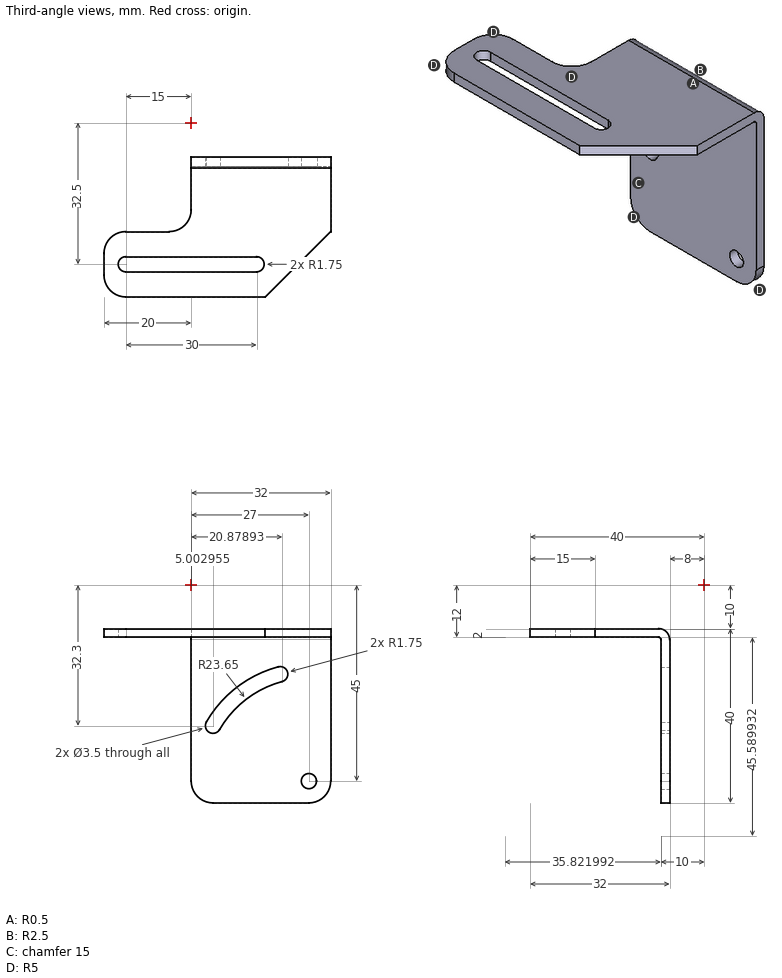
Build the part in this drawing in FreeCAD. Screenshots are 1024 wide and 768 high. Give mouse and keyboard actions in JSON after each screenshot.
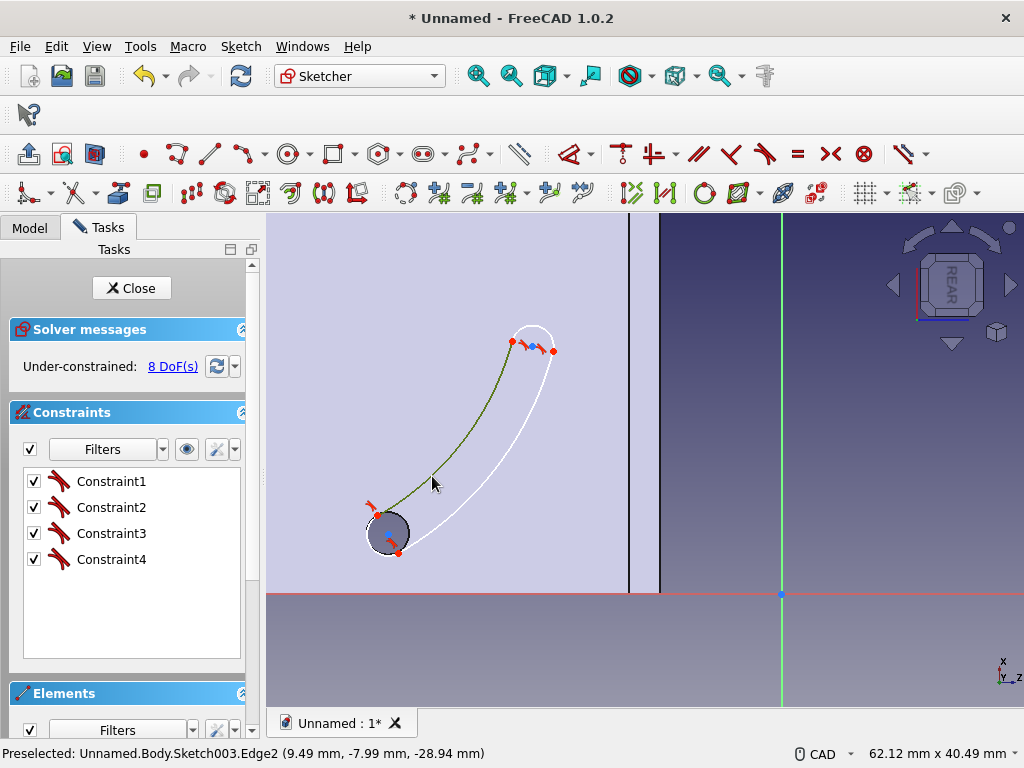
{"action": "left_click", "coordinate": [461, 506]}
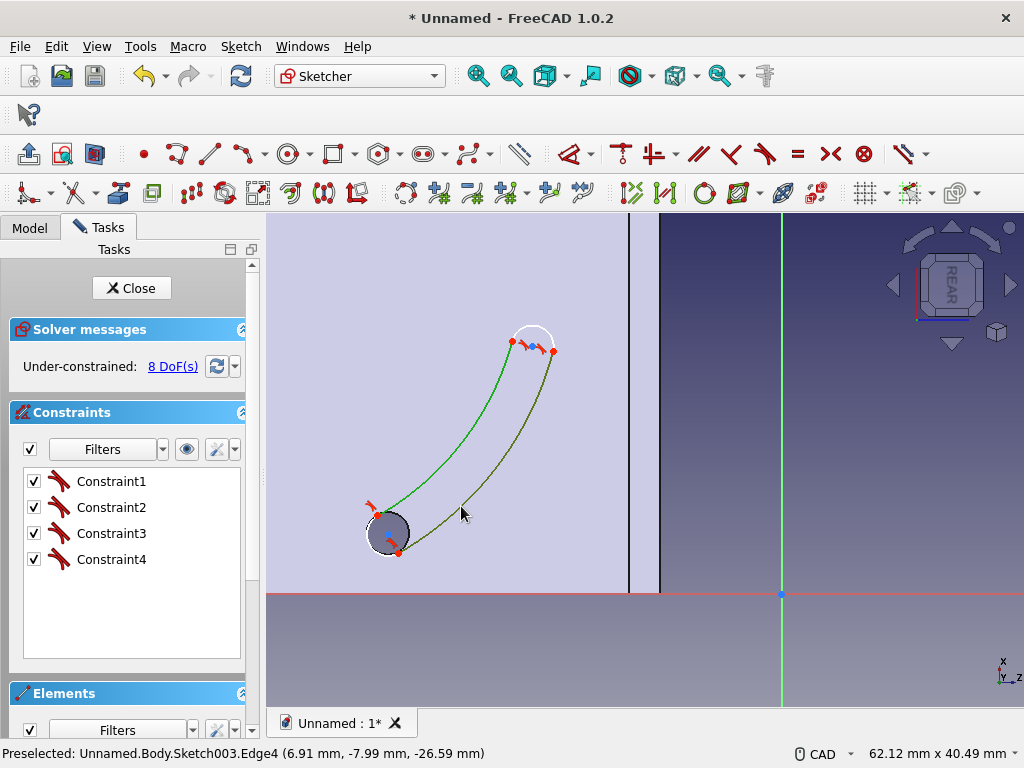
{"action": "key", "text": "c"}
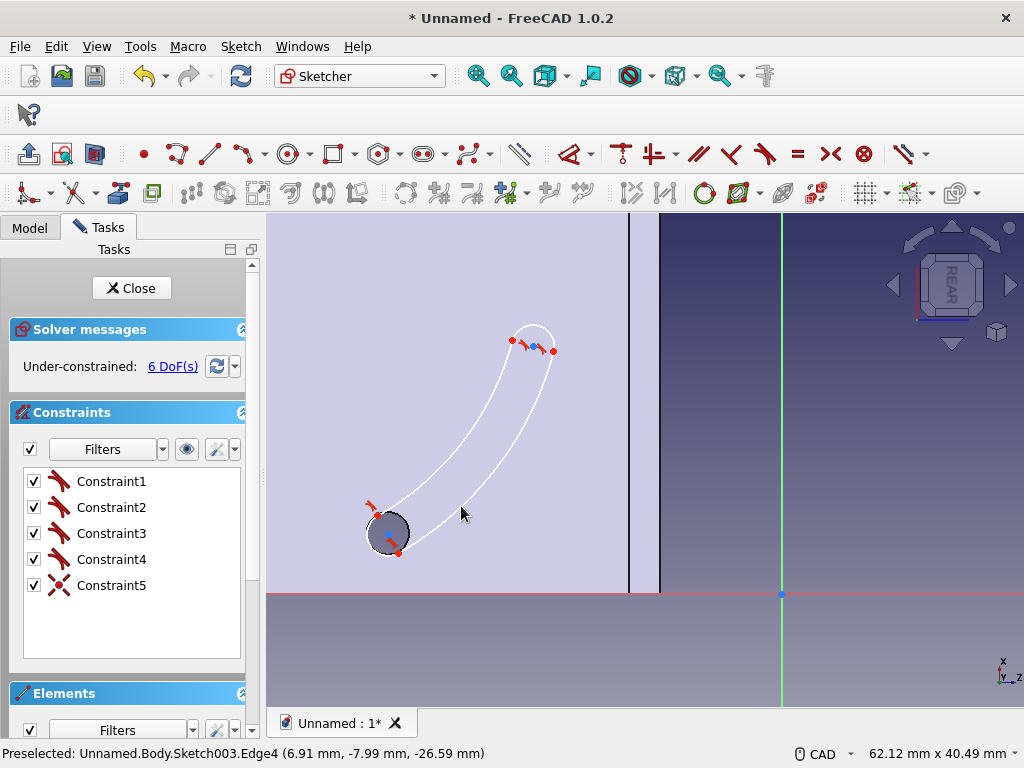
{"action": "key", "text": "d"}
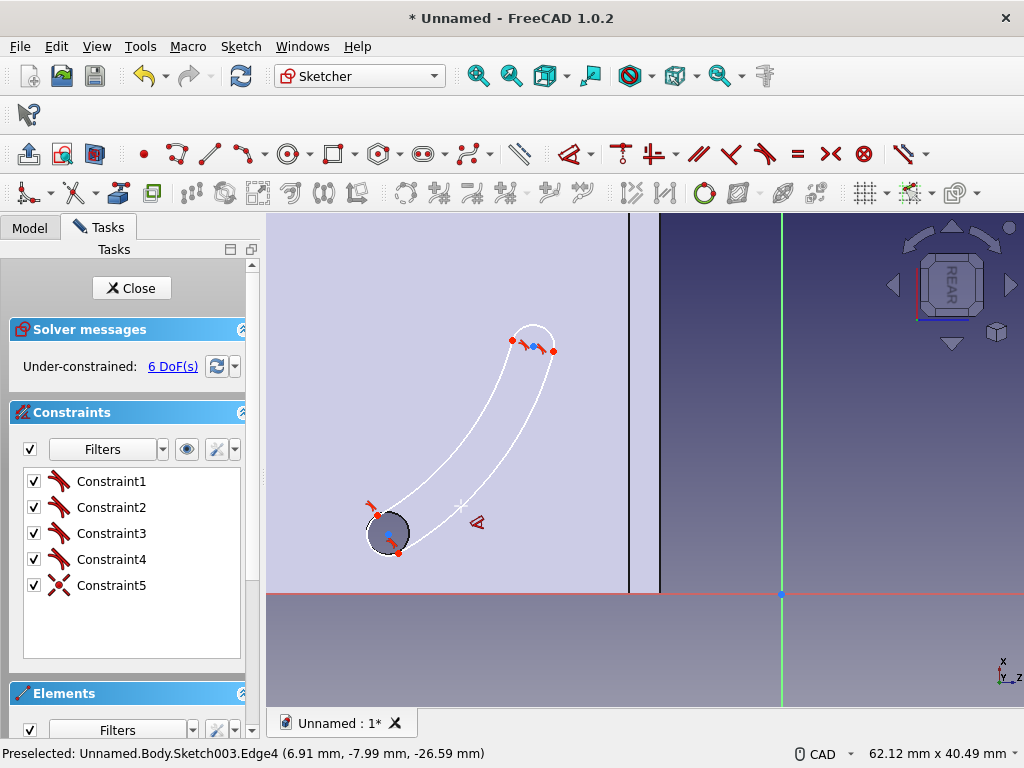
{"action": "scroll", "coordinate": [550, 333], "scroll_direction": "up", "scroll_amount": 4}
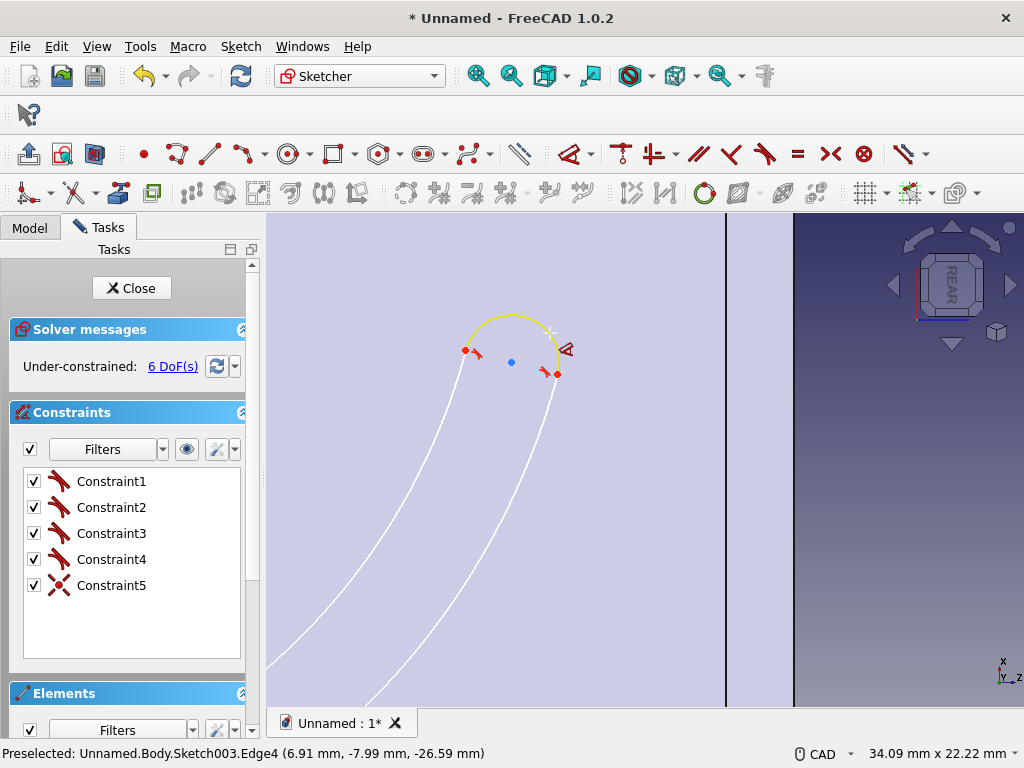
{"action": "left_click", "coordinate": [549, 333]}
{"action": "left_click", "coordinate": [574, 313]}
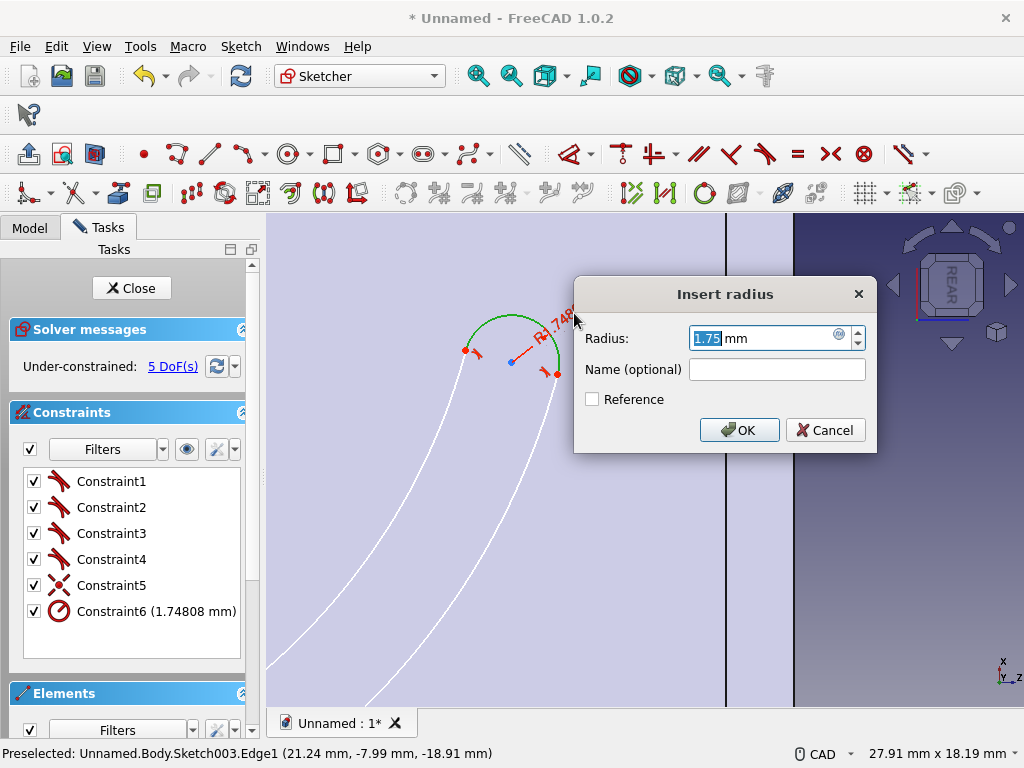
{"action": "type", "text": "1.75"}
{"action": "key", "text": "Return"}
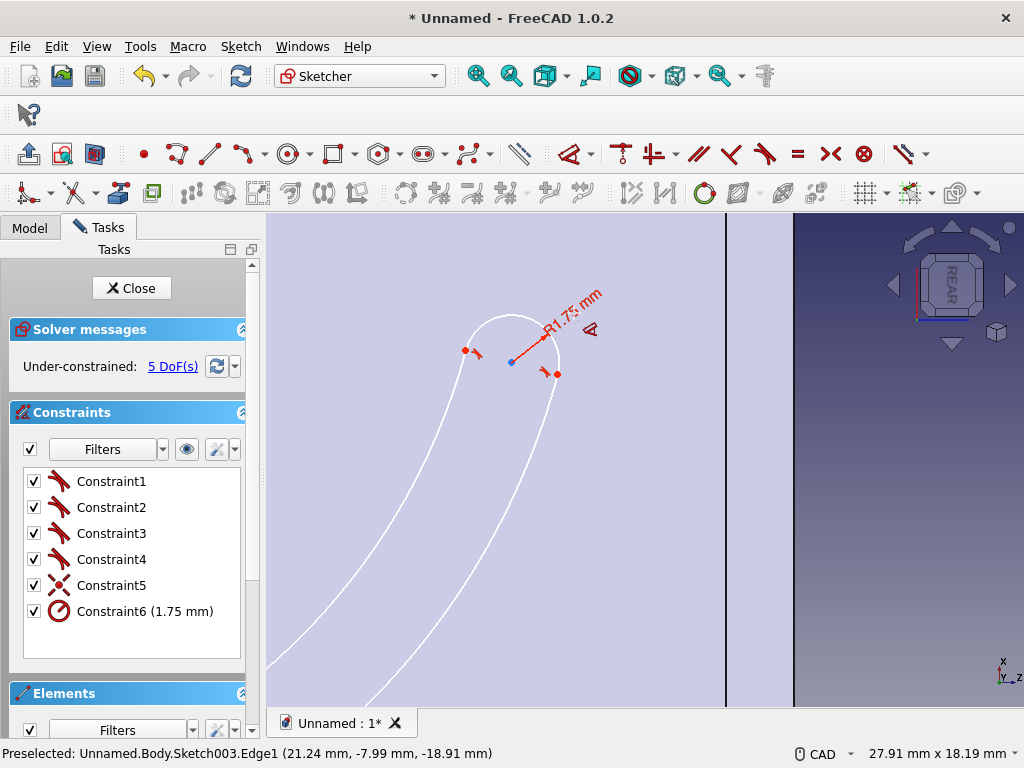
{"action": "left_click", "coordinate": [410, 491]}
{"action": "left_click", "coordinate": [438, 506]}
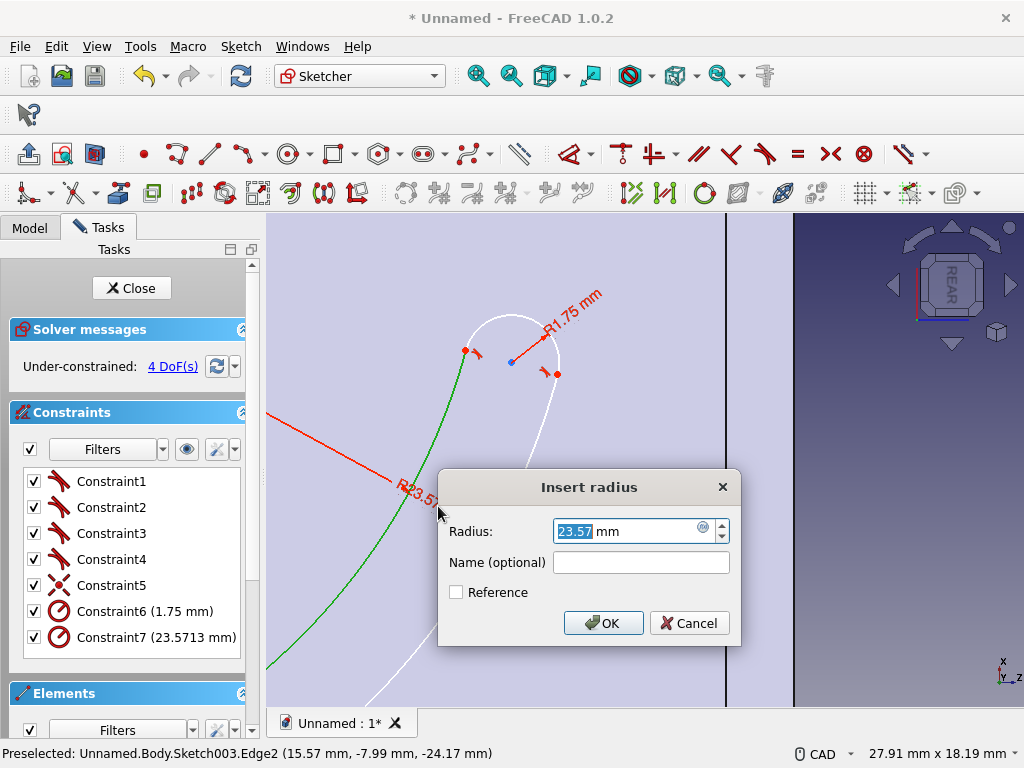
{"action": "type", "text": "23.65"}
{"action": "key", "text": "Return"}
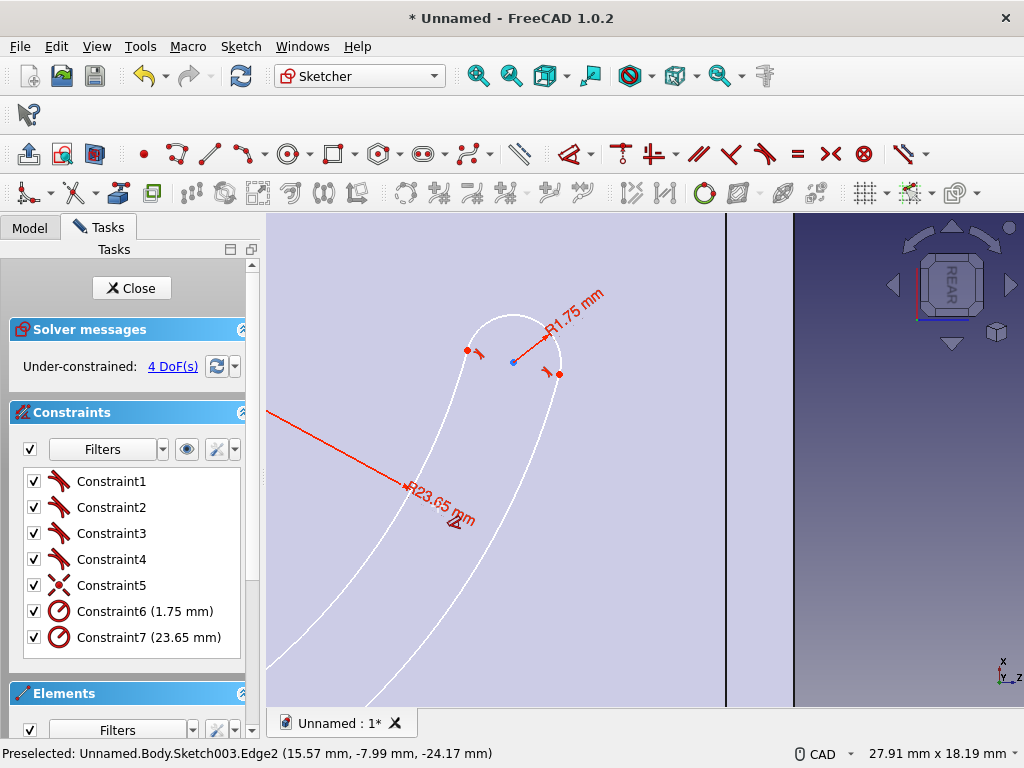
{"action": "scroll", "coordinate": [552, 334], "scroll_direction": "down", "scroll_amount": 4}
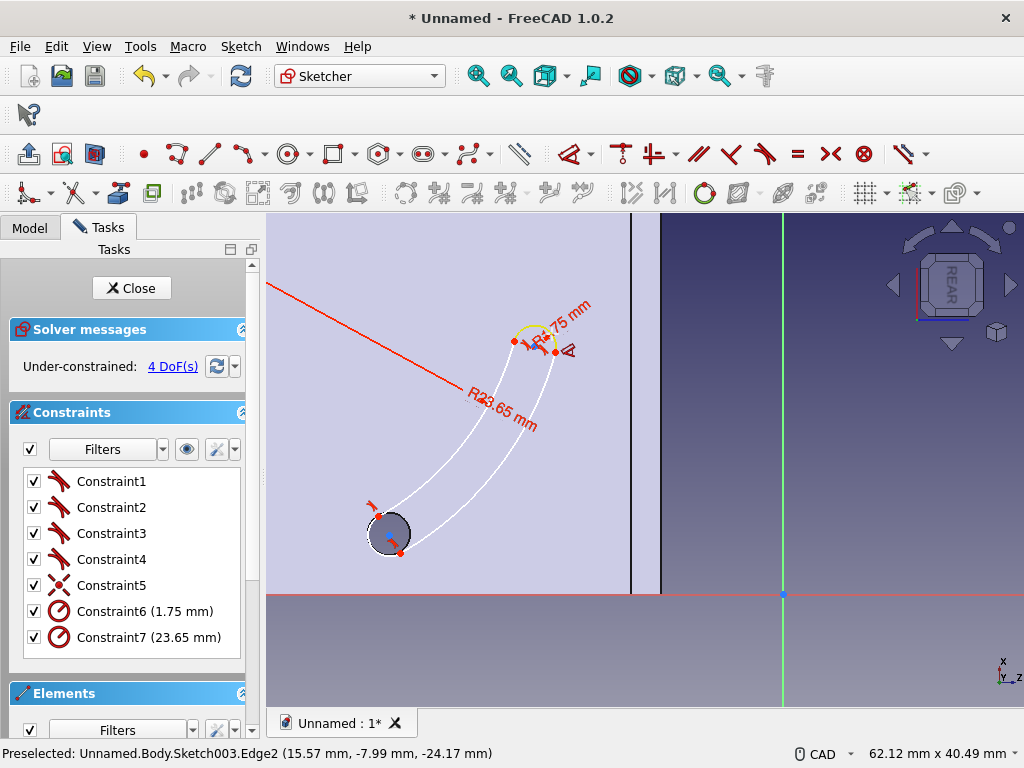
{"action": "scroll", "coordinate": [713, 520], "scroll_direction": "down", "scroll_amount": 2}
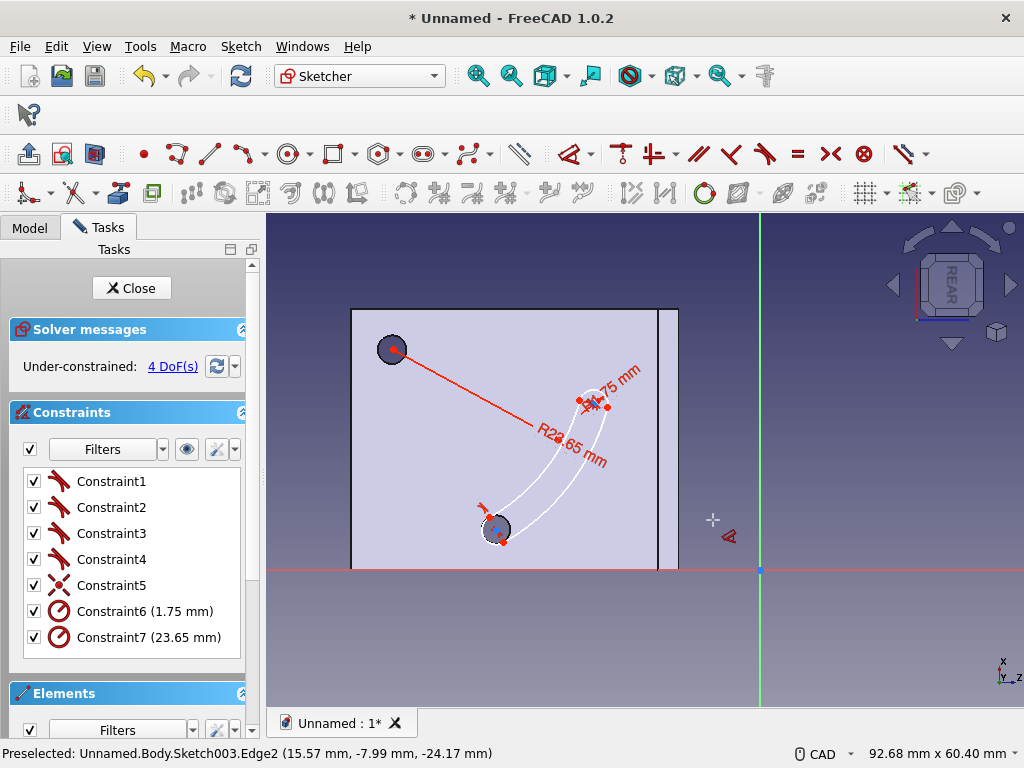
{"action": "left_click", "coordinate": [393, 350]}
{"action": "left_click", "coordinate": [577, 316]}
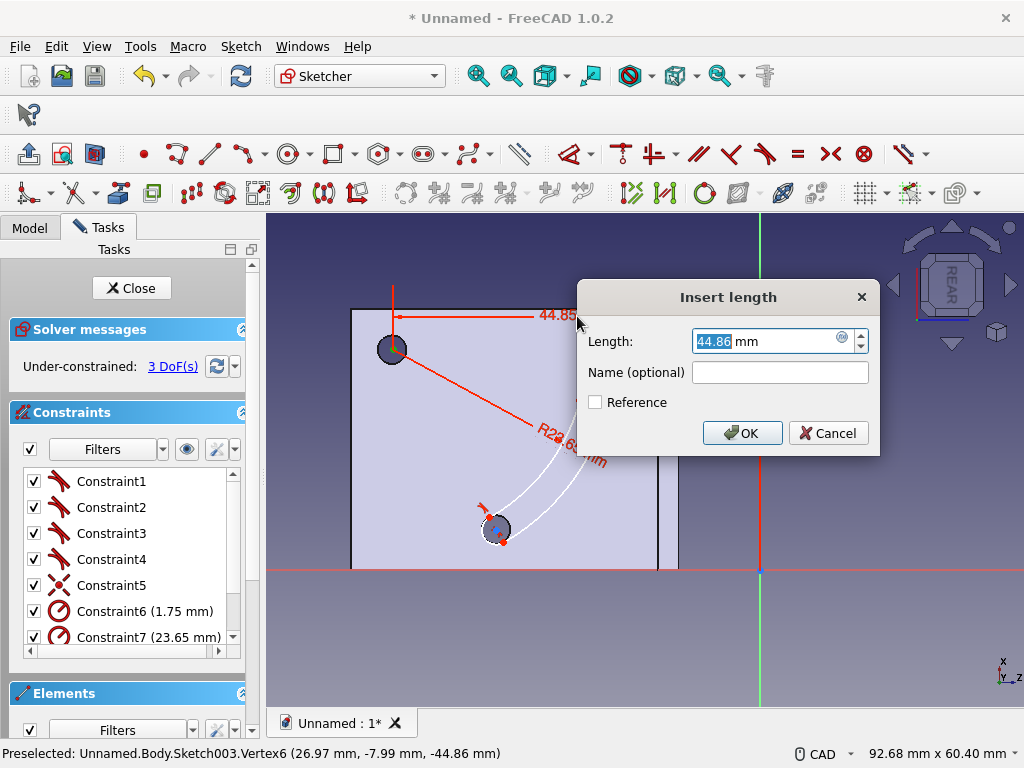
{"action": "type", "text": "45"}
{"action": "key", "text": "Return"}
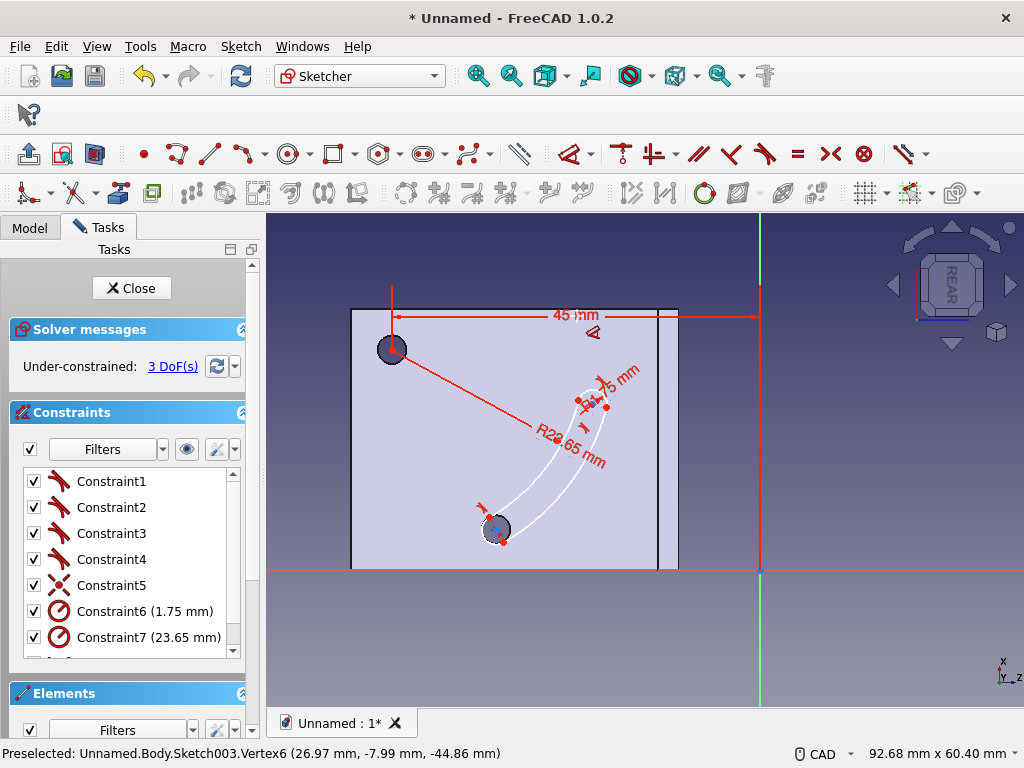
{"action": "left_click", "coordinate": [392, 351]}
{"action": "left_click", "coordinate": [358, 461]}